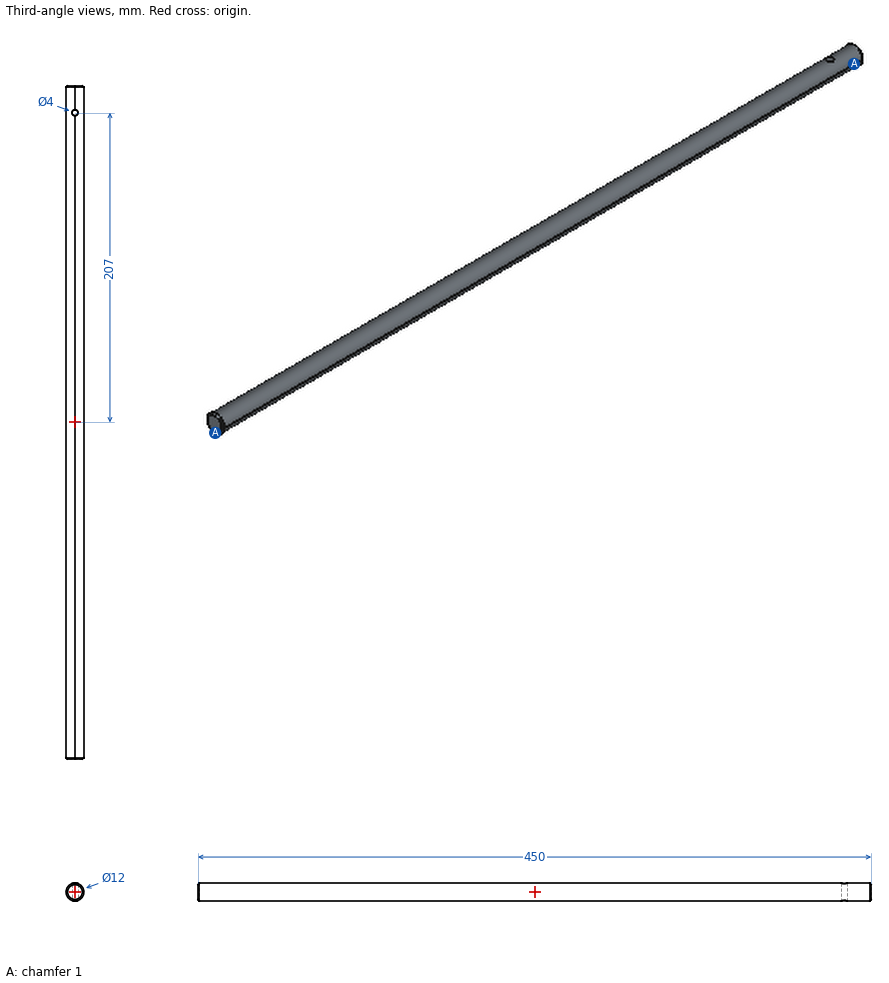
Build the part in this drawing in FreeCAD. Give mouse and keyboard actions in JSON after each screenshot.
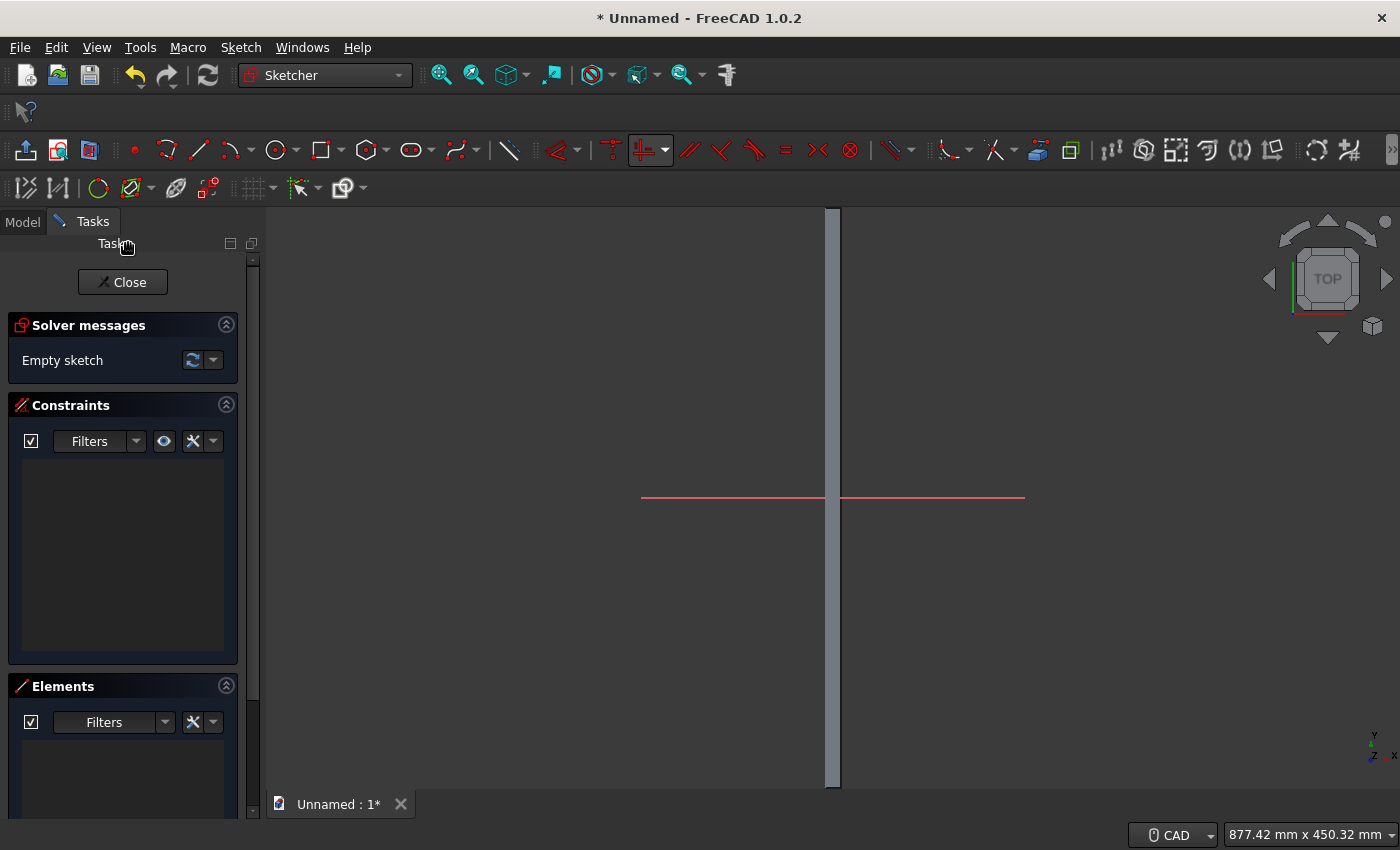
{"action": "key", "text": "q s"}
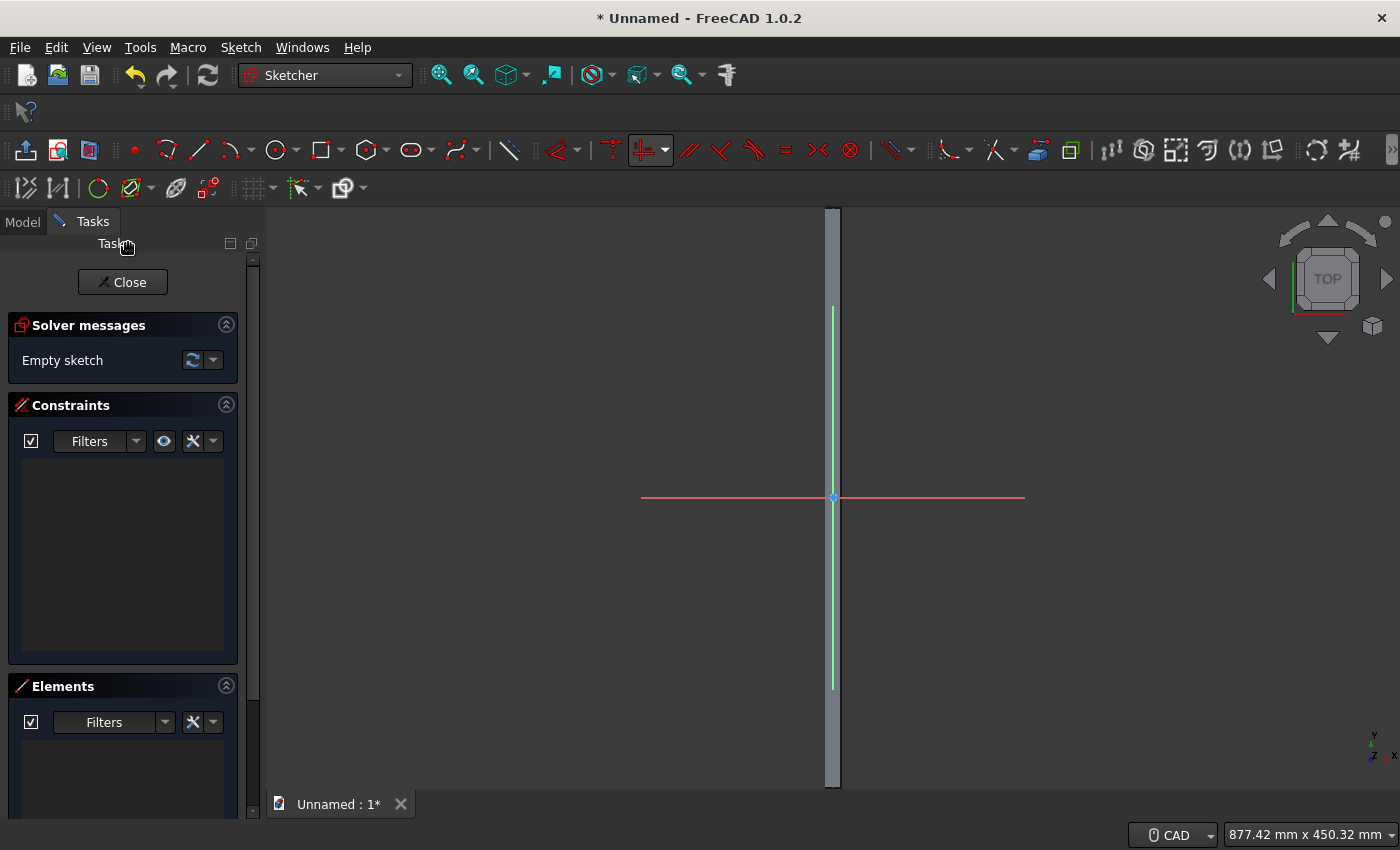
{"action": "scroll", "coordinate": [764, 498], "scroll_direction": "down", "scroll_amount": 5}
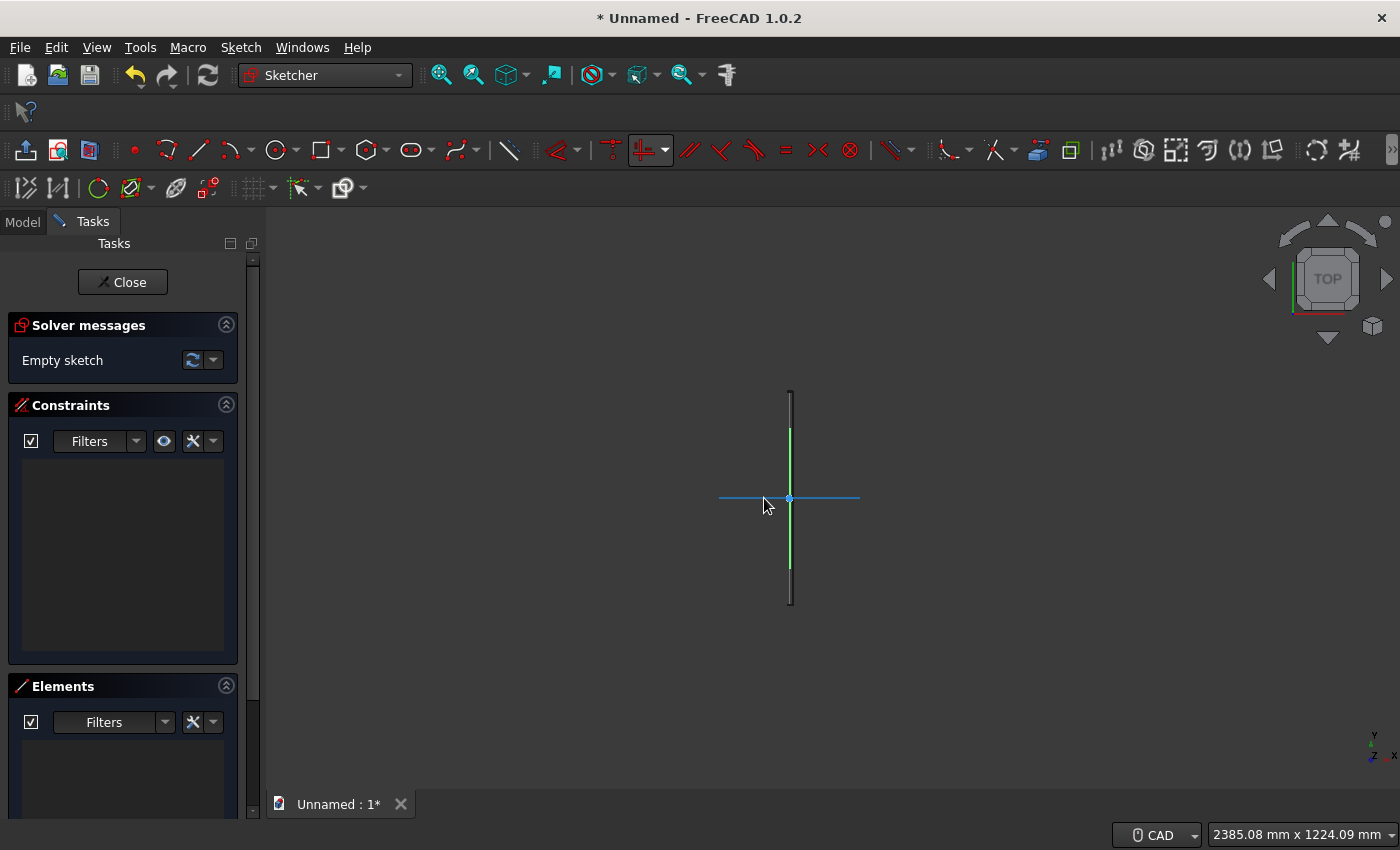
{"action": "scroll", "coordinate": [791, 395], "scroll_direction": "up", "scroll_amount": 15}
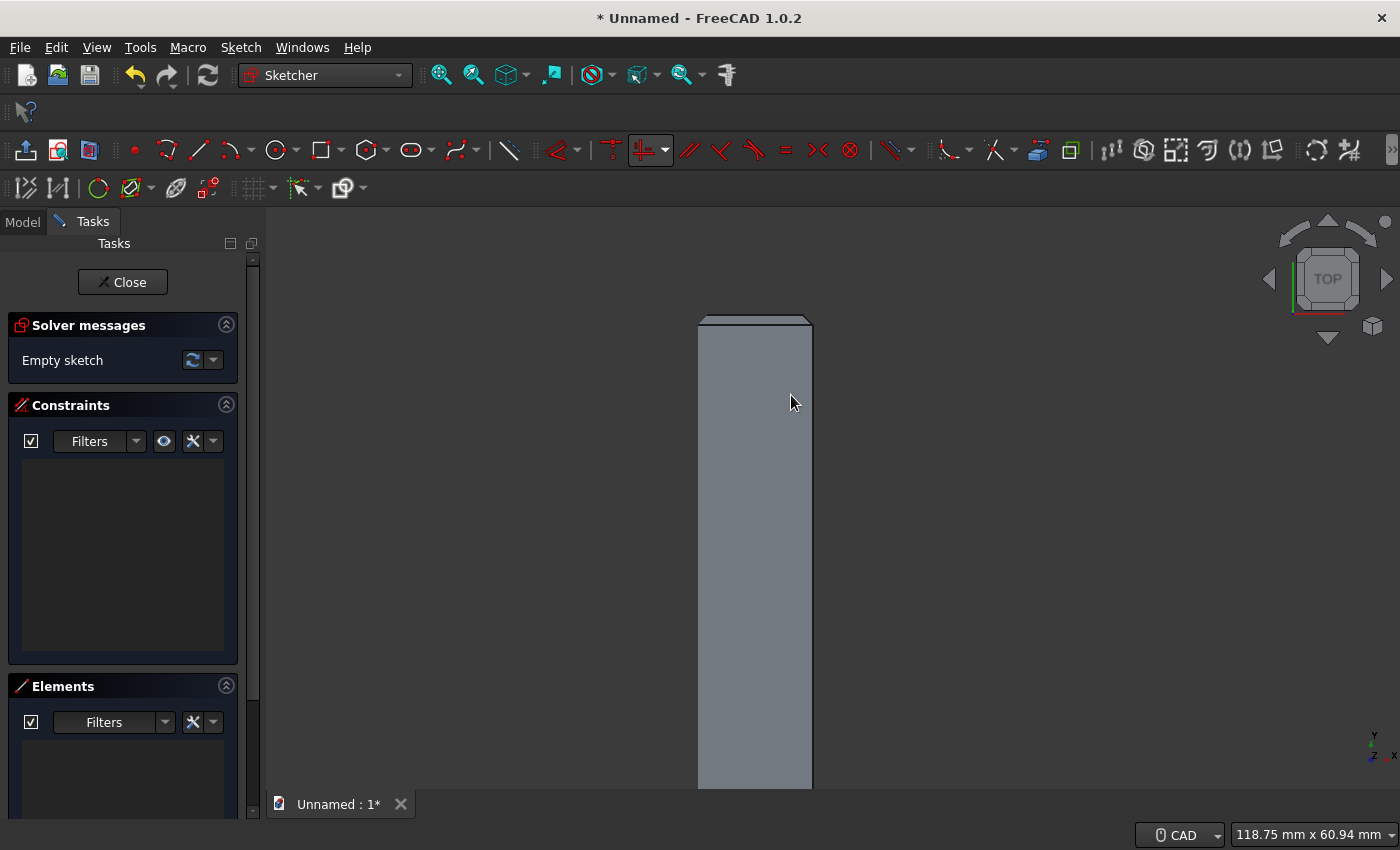
{"action": "scroll", "coordinate": [754, 486], "scroll_direction": "up", "scroll_amount": 11}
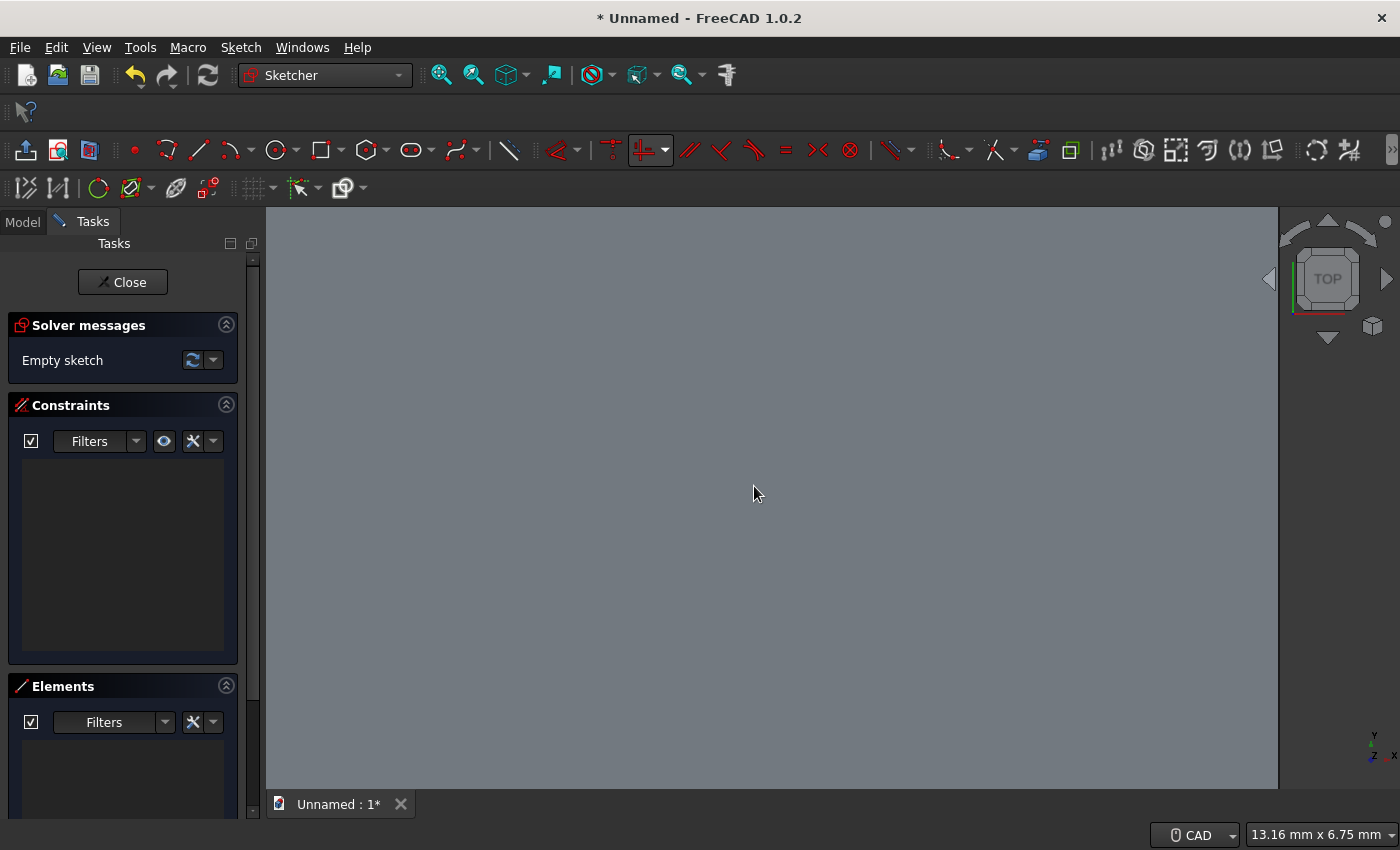
{"action": "key", "text": "g c"}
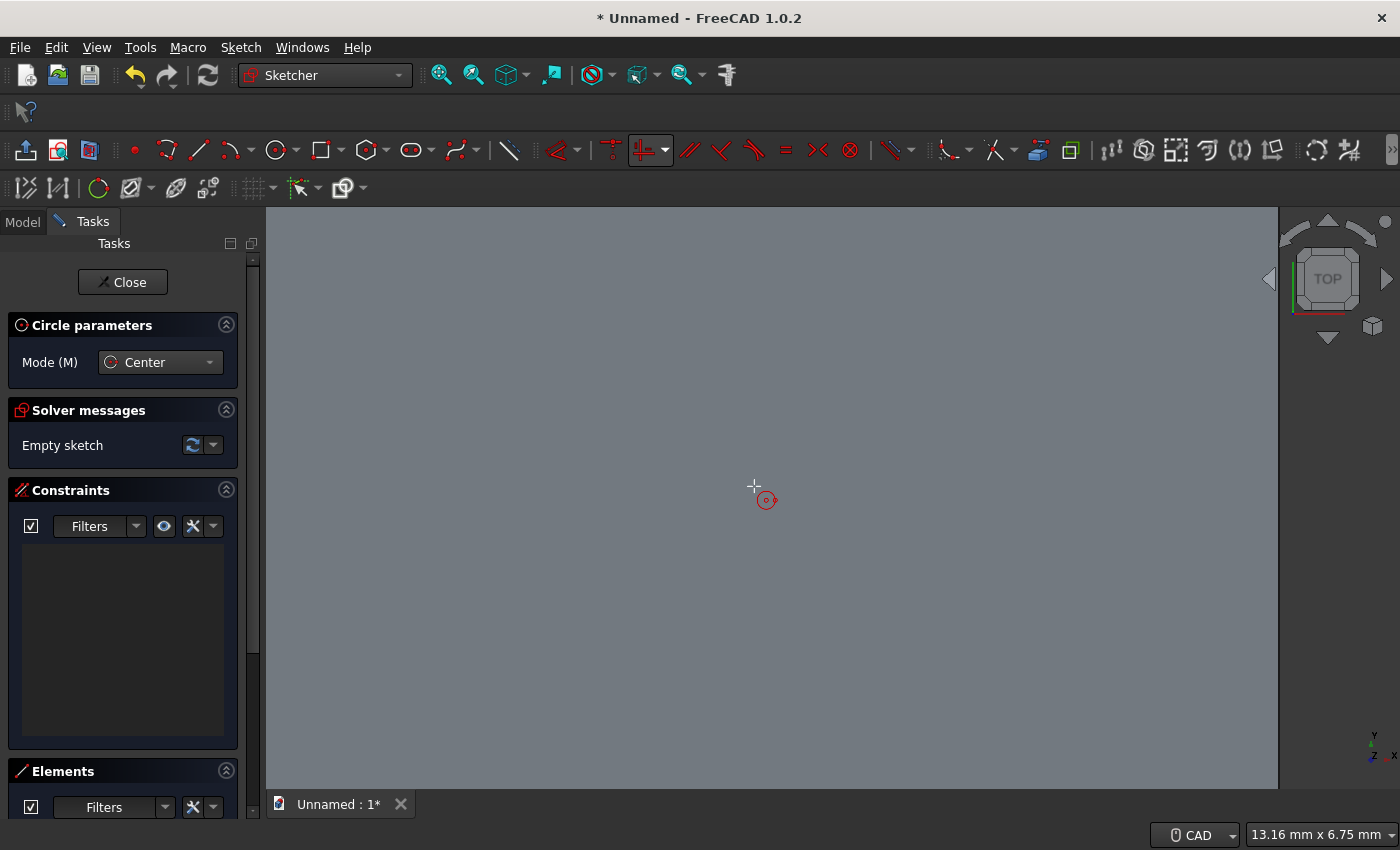
{"action": "left_click", "coordinate": [762, 493]}
{"action": "left_click", "coordinate": [884, 371]}
{"action": "key", "text": "Escape"}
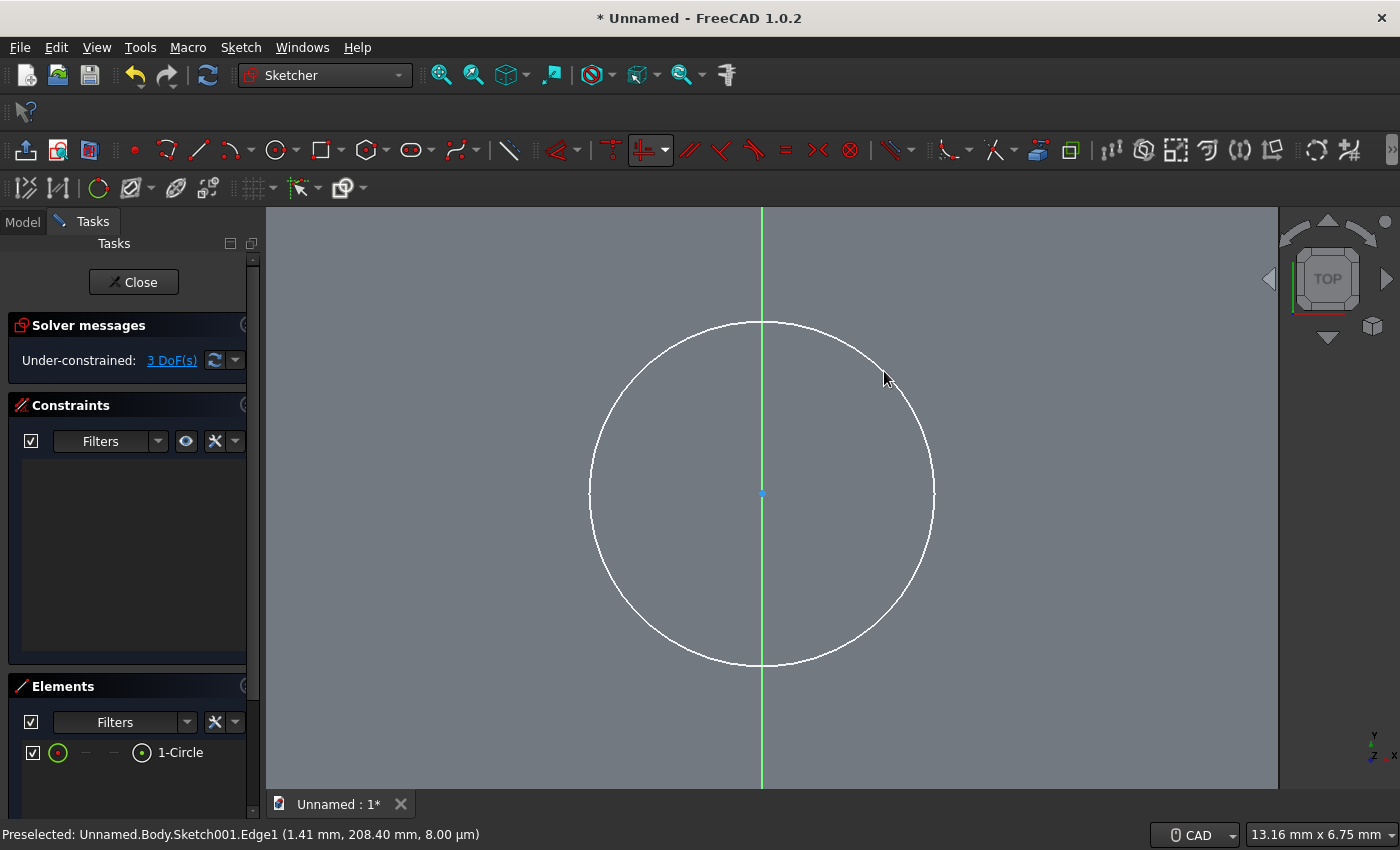
{"action": "left_click", "coordinate": [762, 494]}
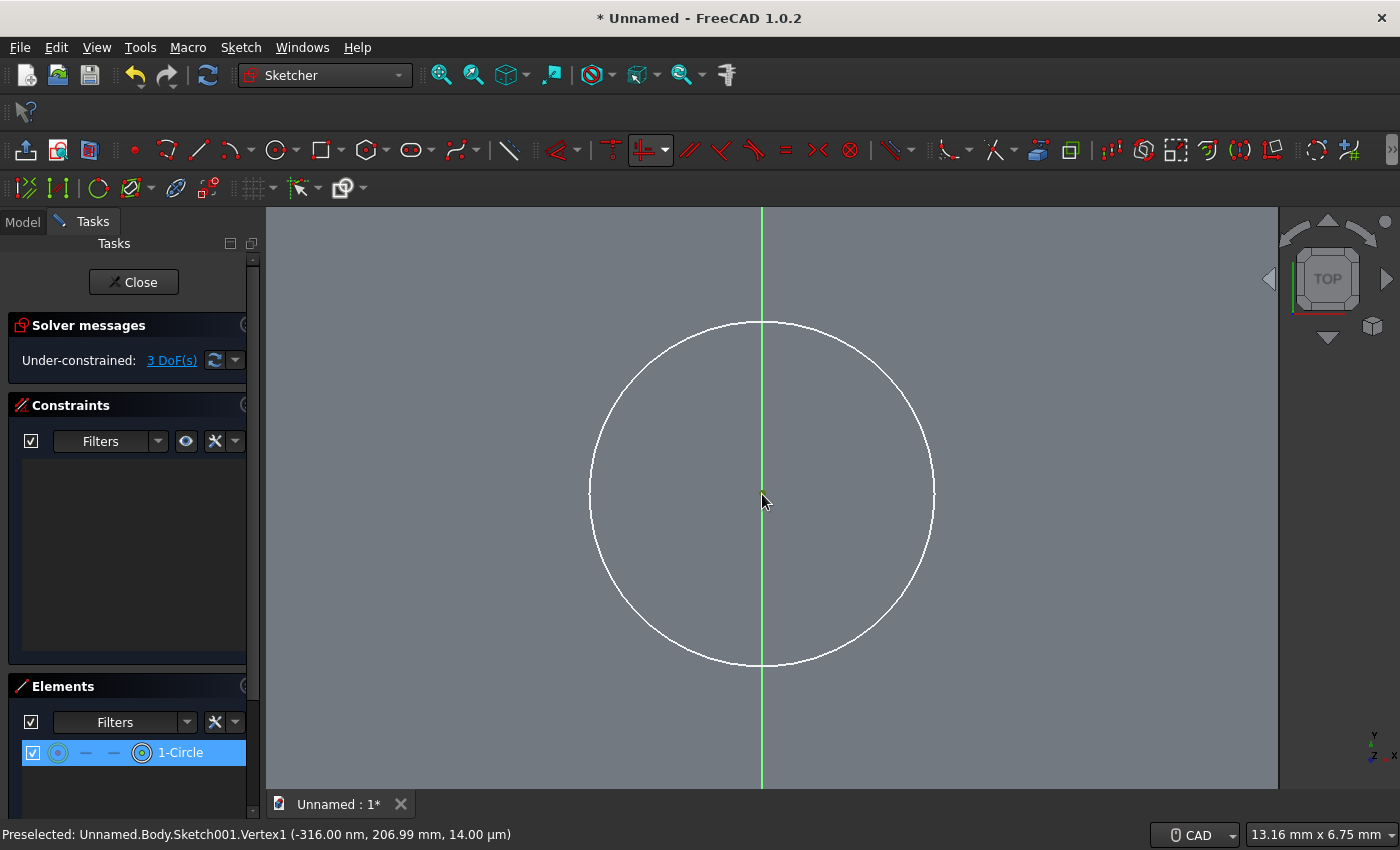
{"action": "left_click", "coordinate": [762, 723]}